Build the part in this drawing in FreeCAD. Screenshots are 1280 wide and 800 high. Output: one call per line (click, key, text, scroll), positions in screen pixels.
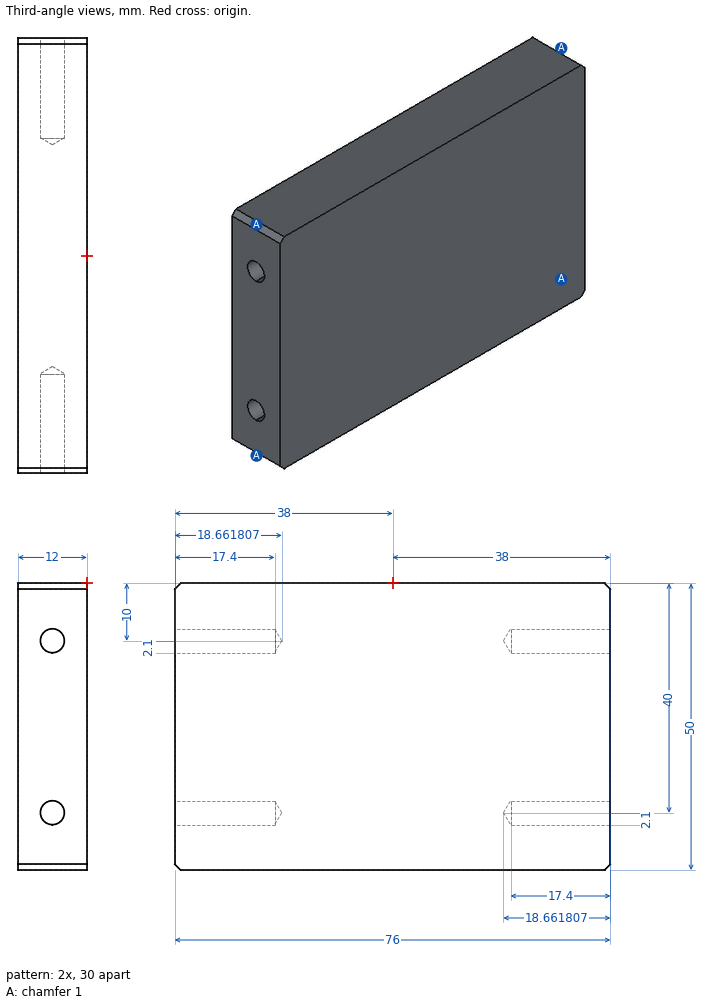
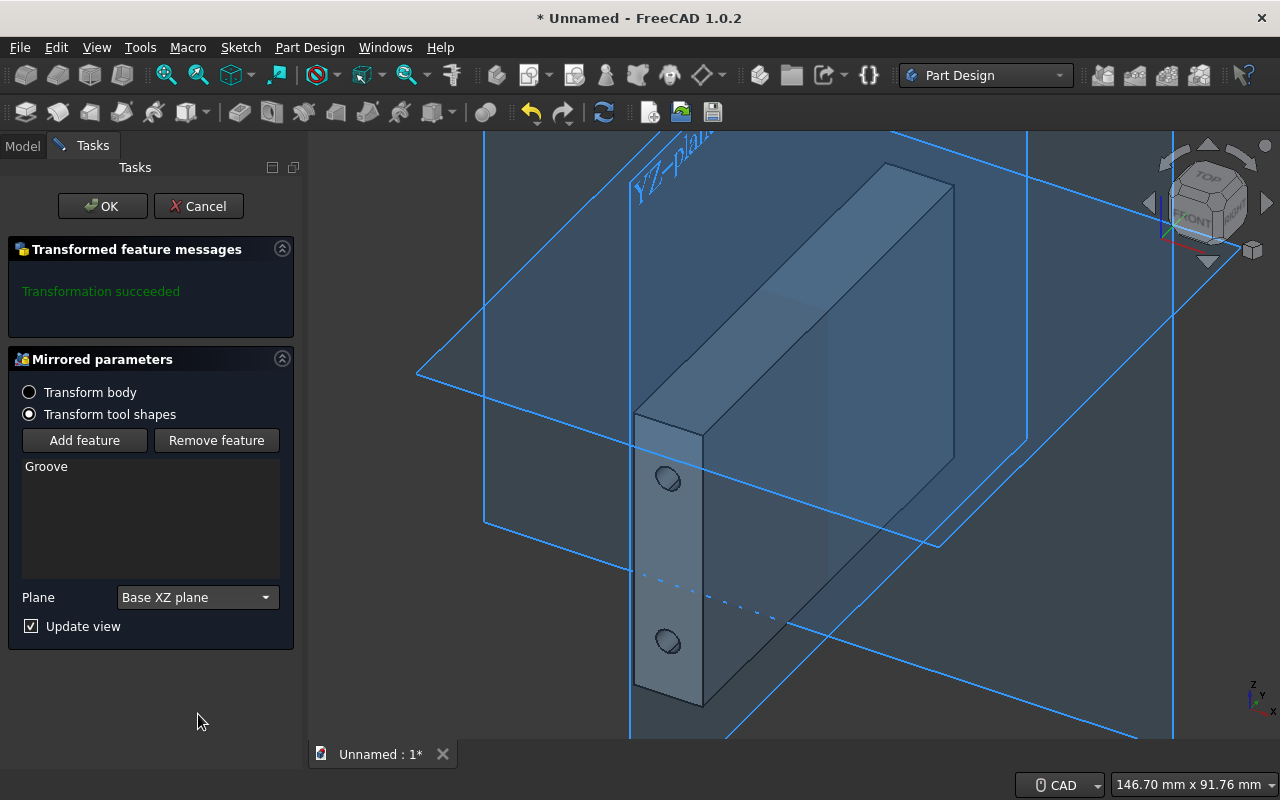
click(103, 206)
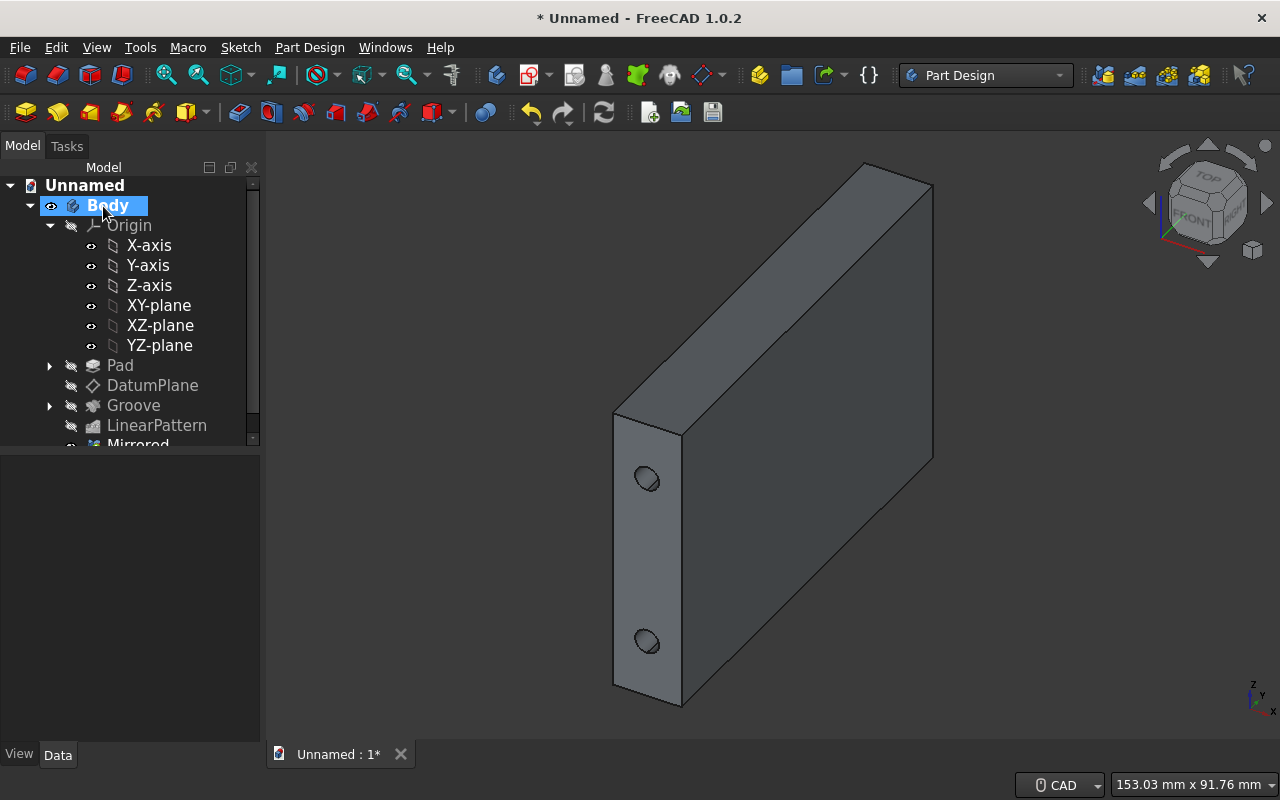
click(136, 346)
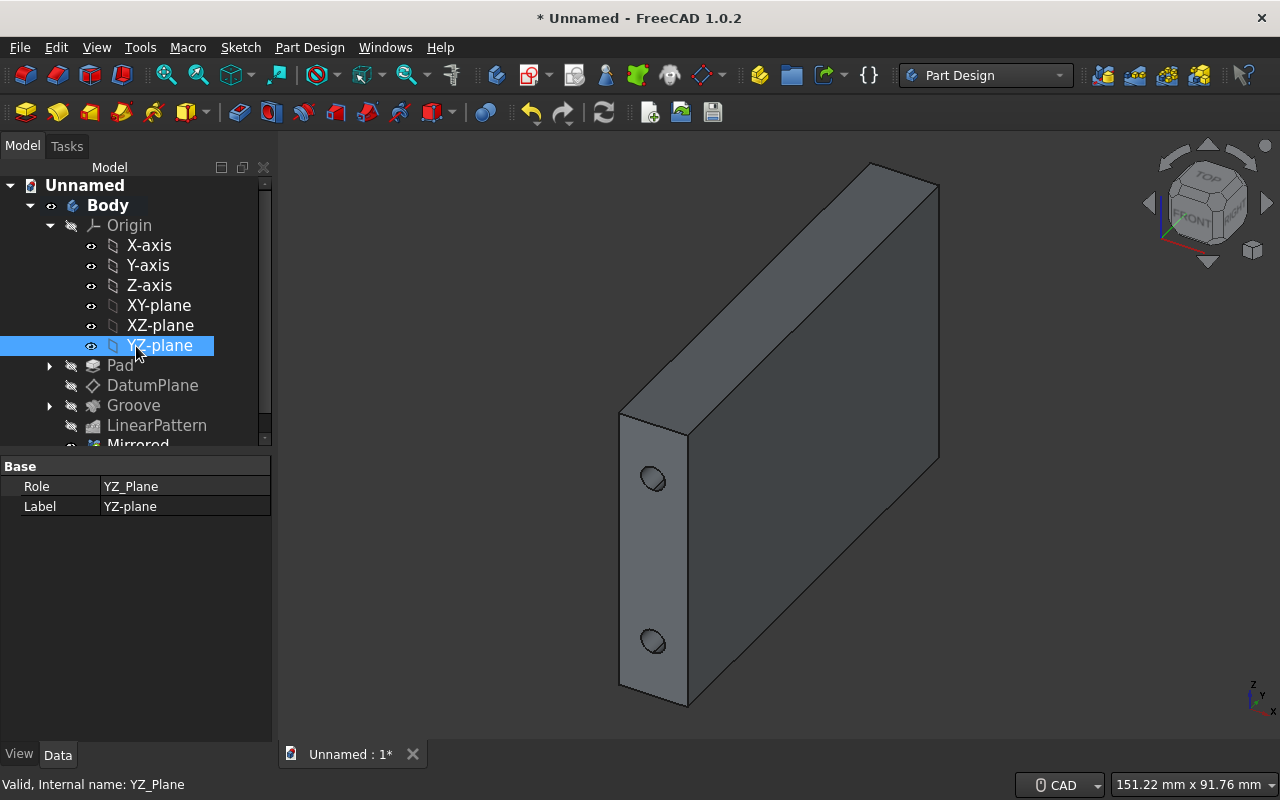
click(702, 76)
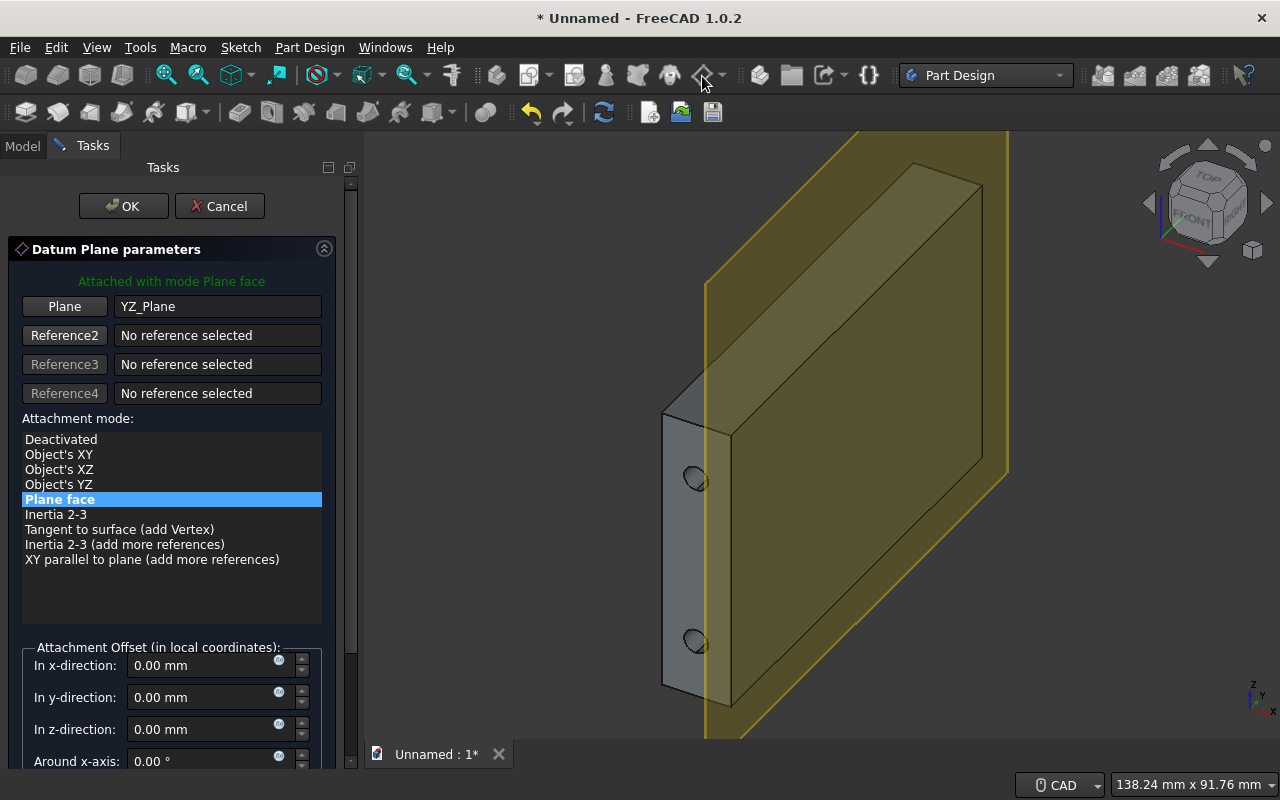
triple_click(210, 729)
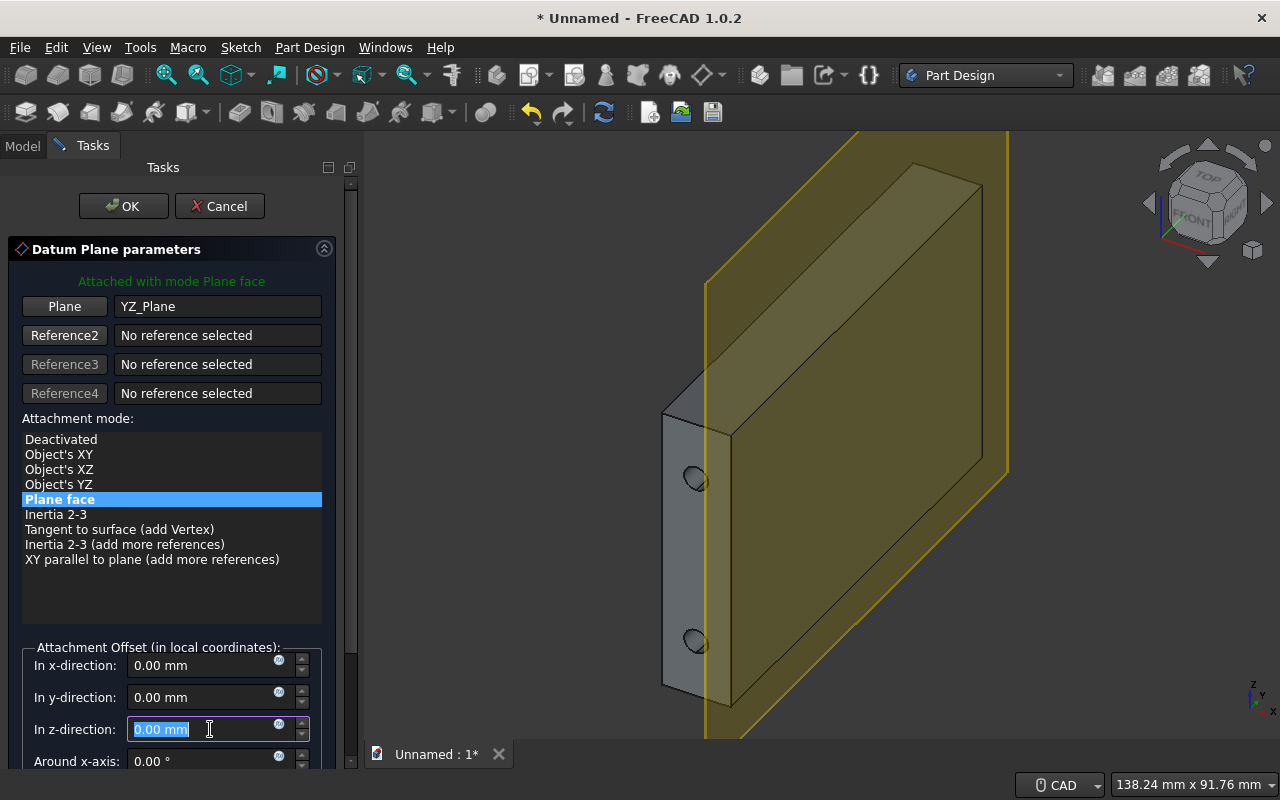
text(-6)
key(Tab)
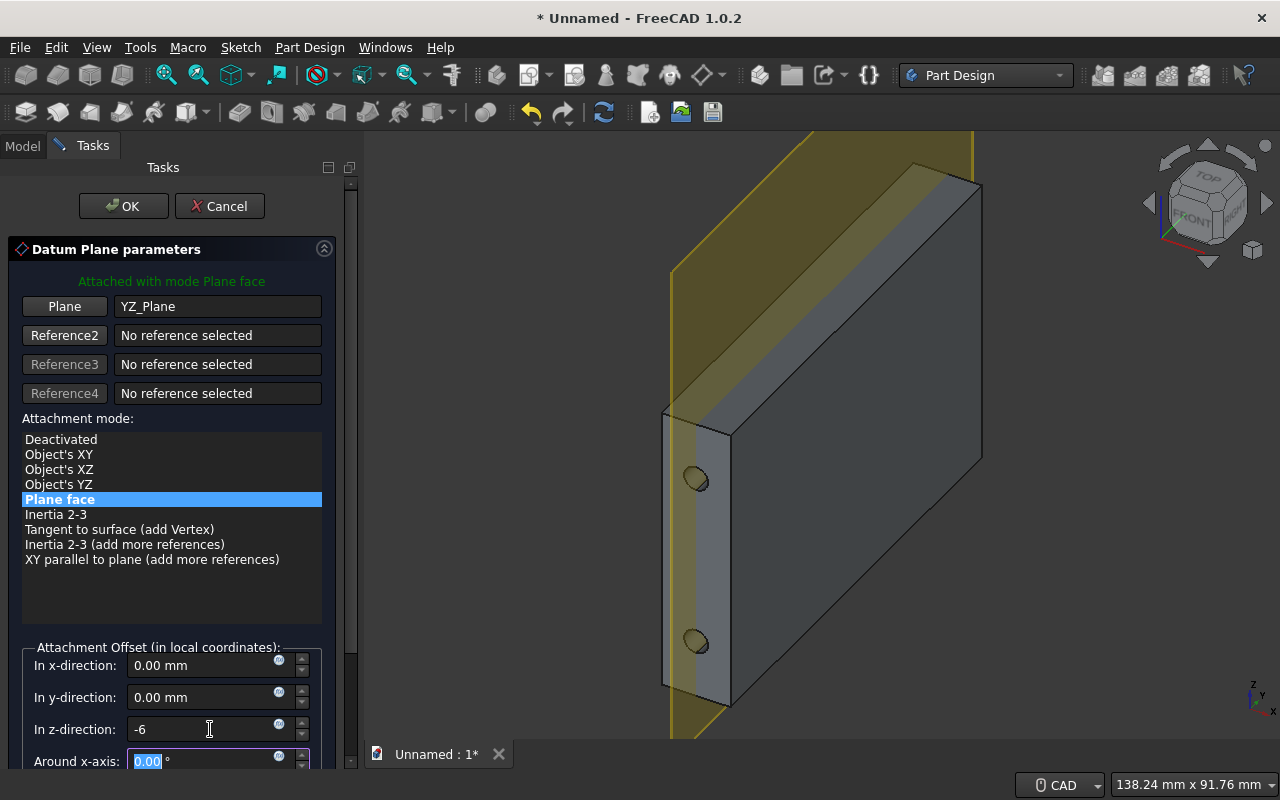
click(124, 206)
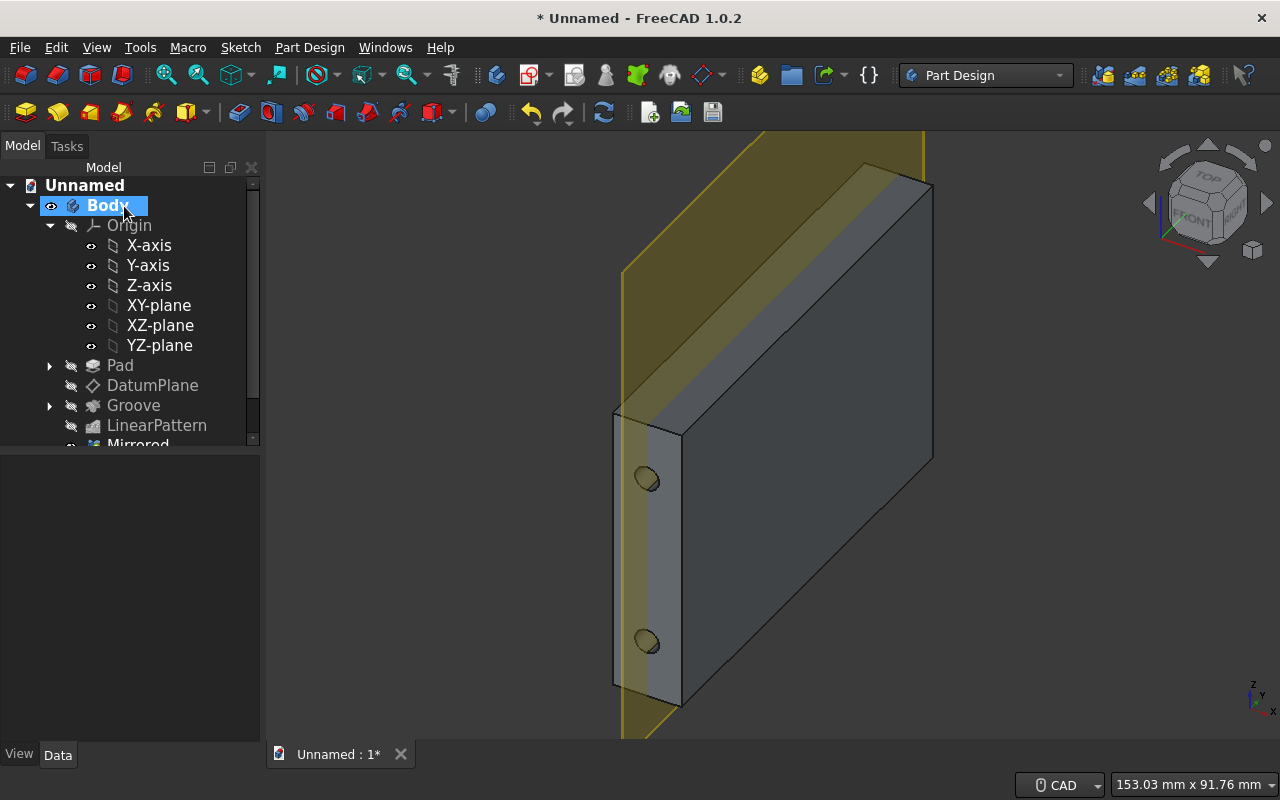
scroll(100, 321, down, 3)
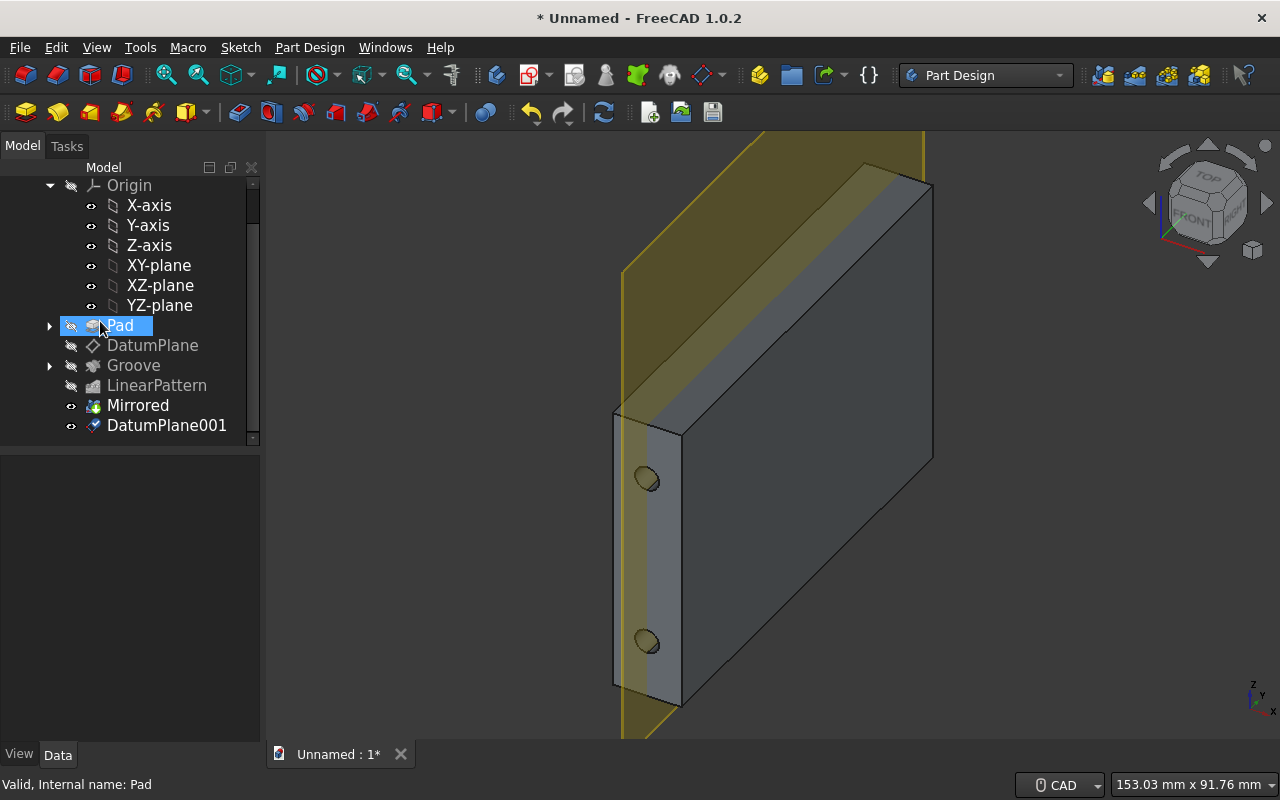
click(116, 426)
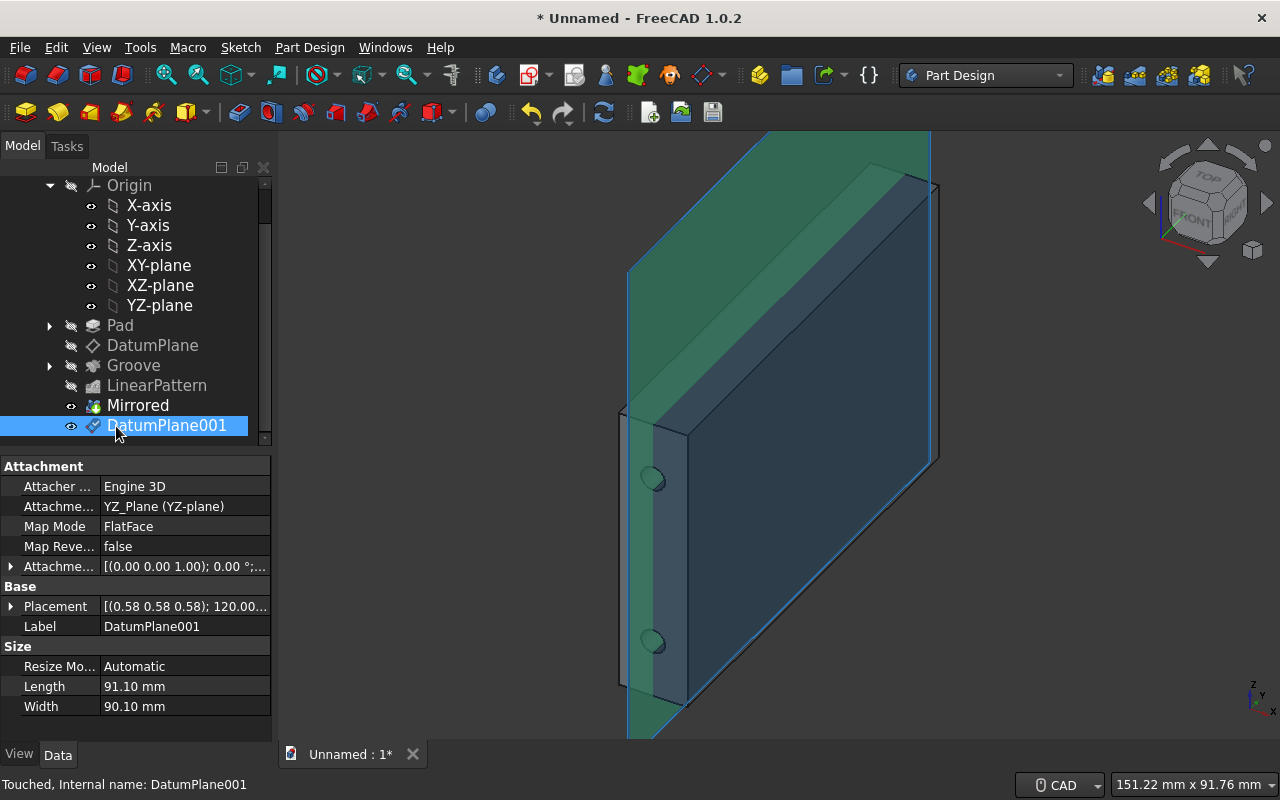
click(530, 76)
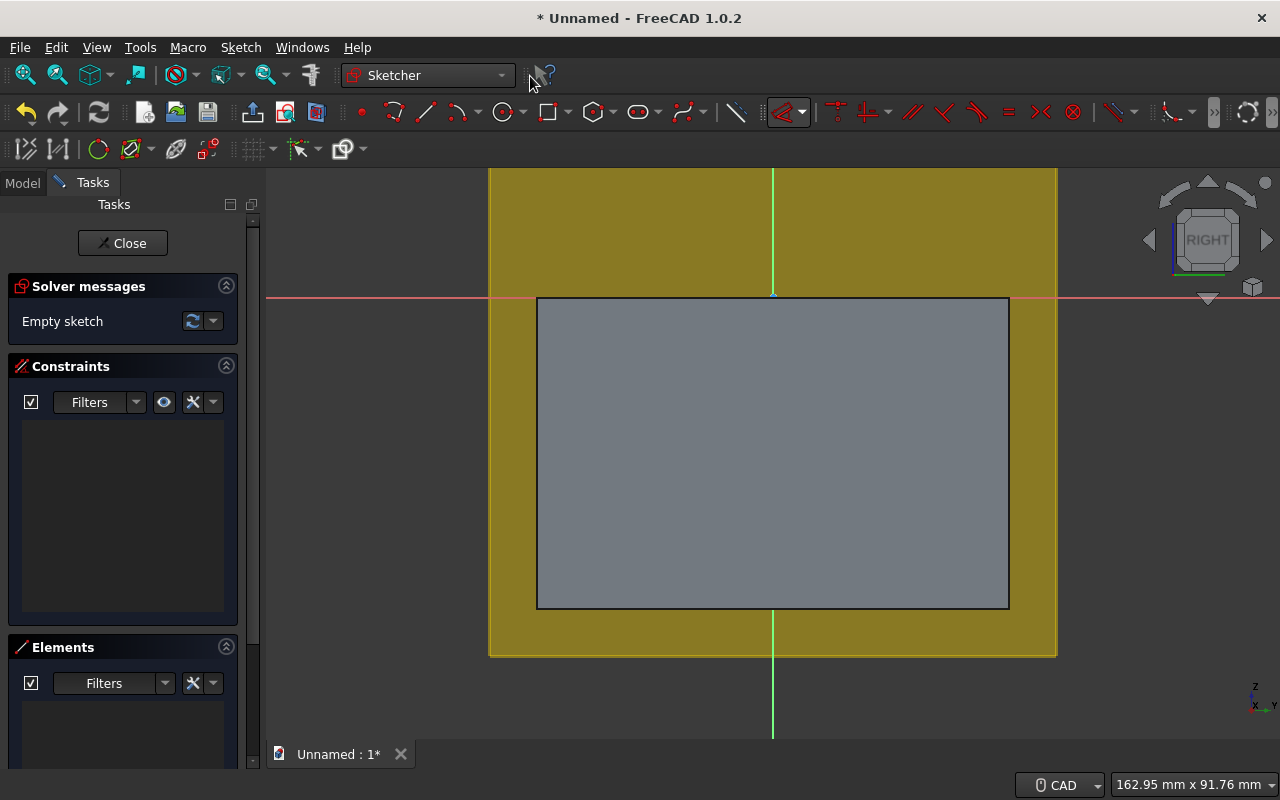
click(318, 112)